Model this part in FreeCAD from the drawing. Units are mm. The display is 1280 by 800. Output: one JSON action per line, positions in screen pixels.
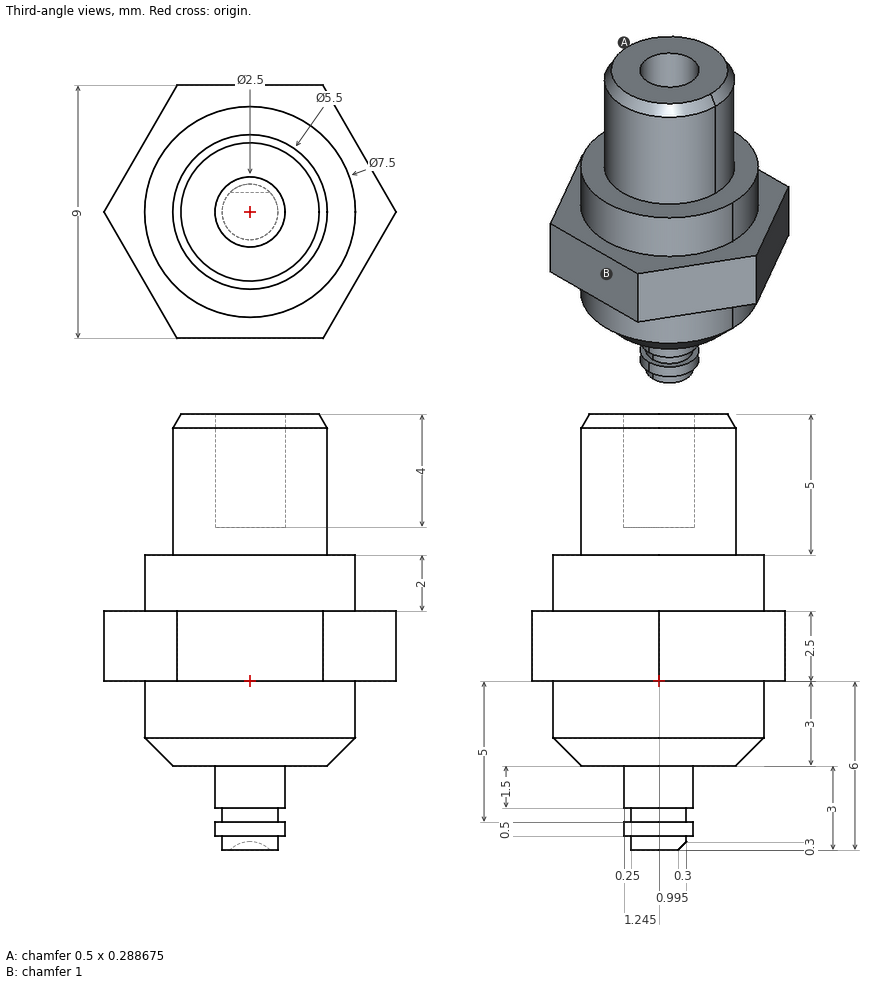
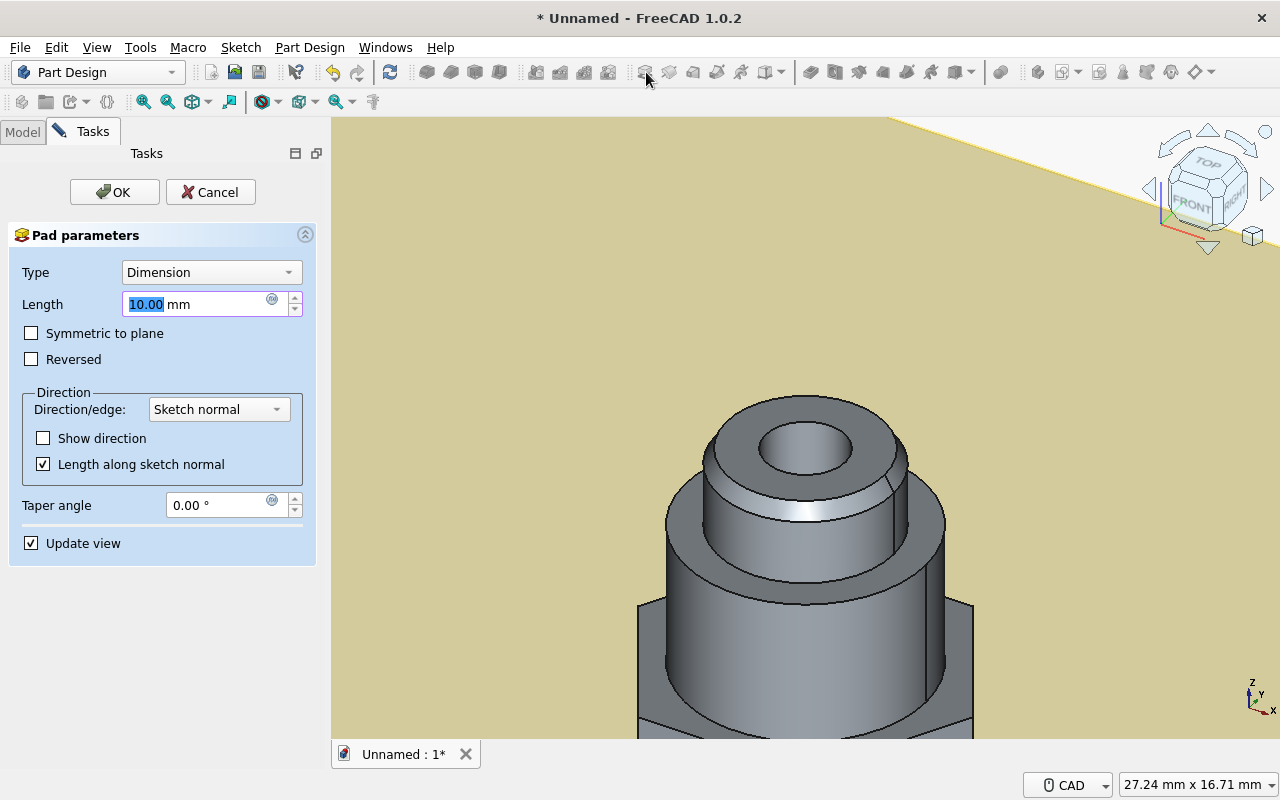
{"action": "type", "text": "3"}
{"action": "key", "text": "Tab"}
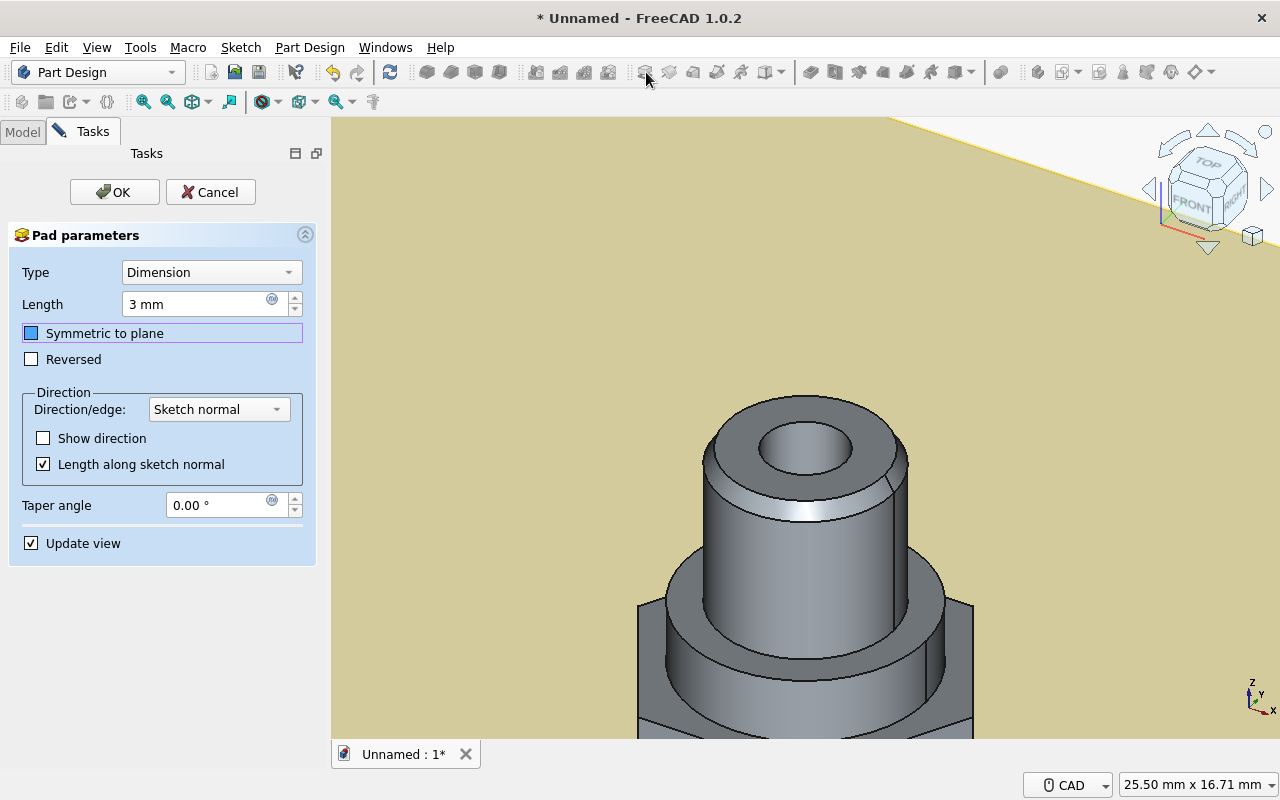
{"action": "left_click", "coordinate": [115, 192]}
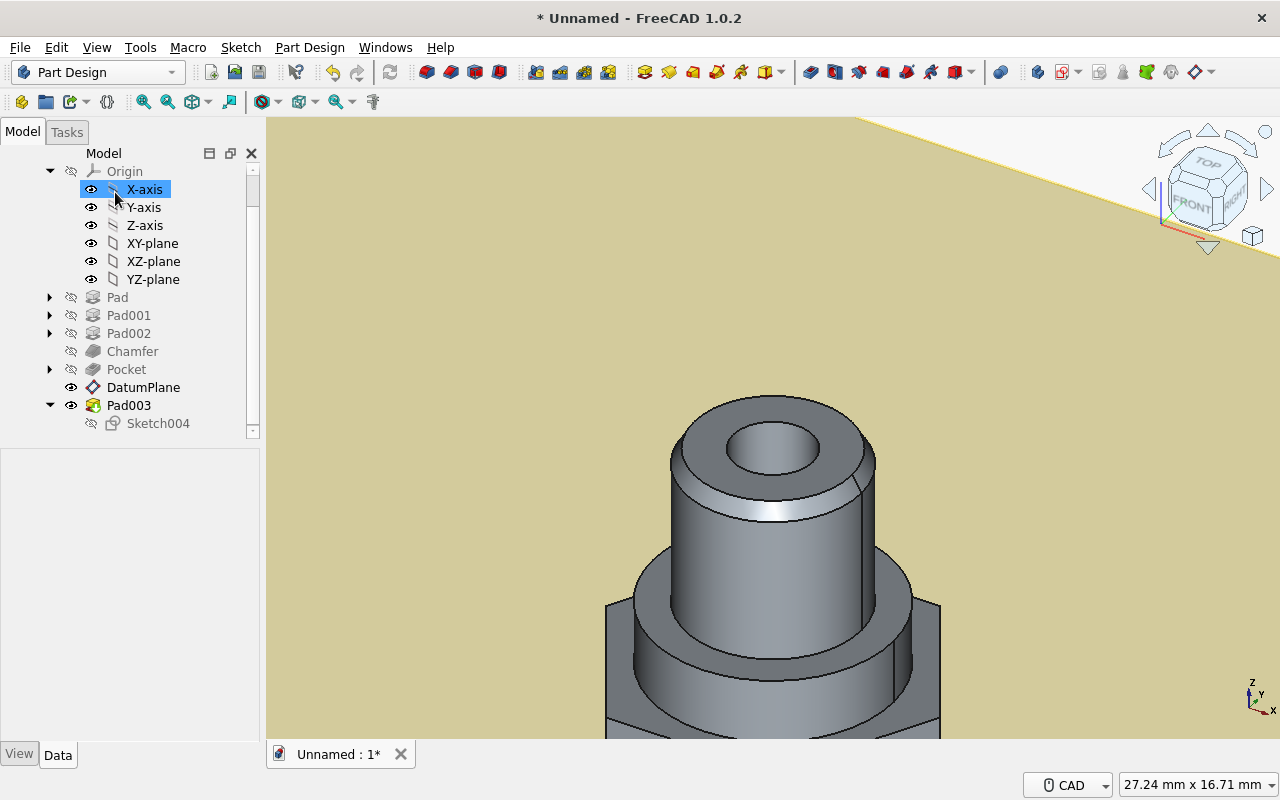
{"action": "left_click", "coordinate": [116, 387]}
{"action": "key", "text": "space"}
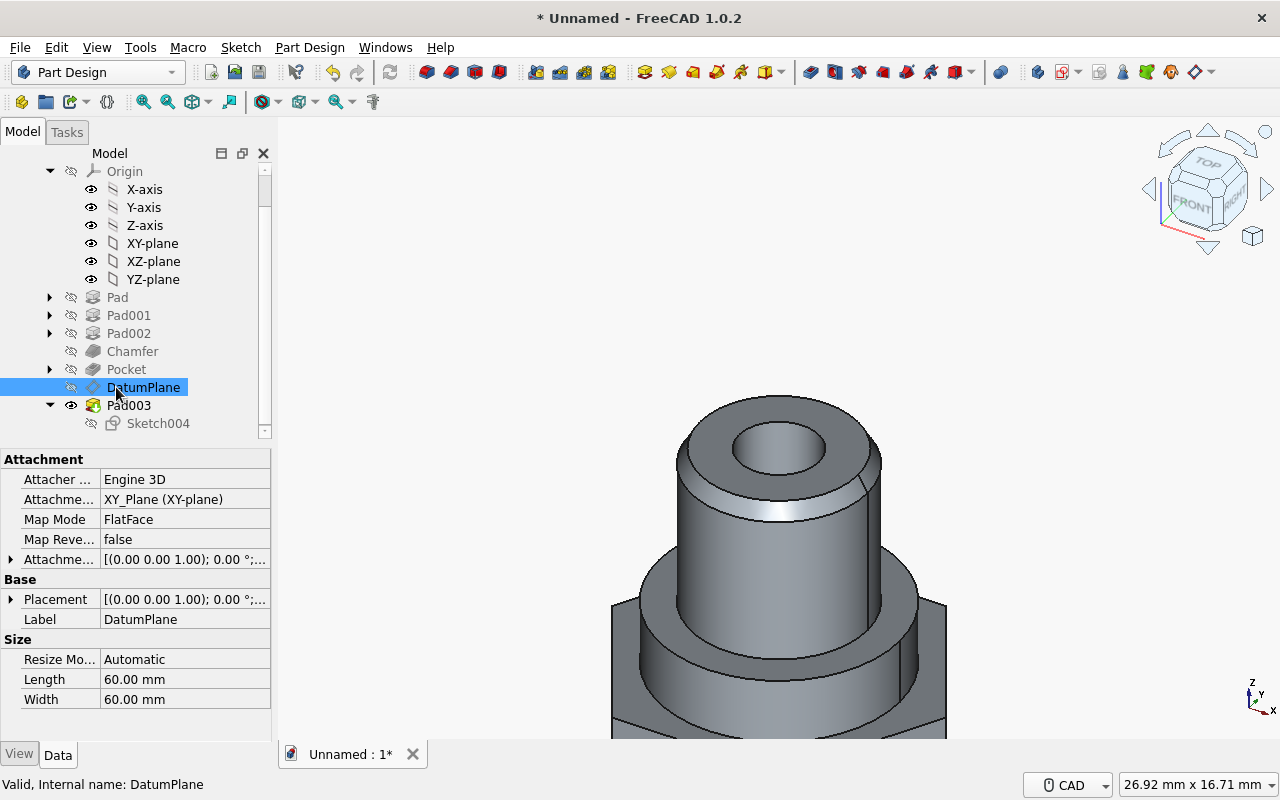
{"action": "key", "text": "v f"}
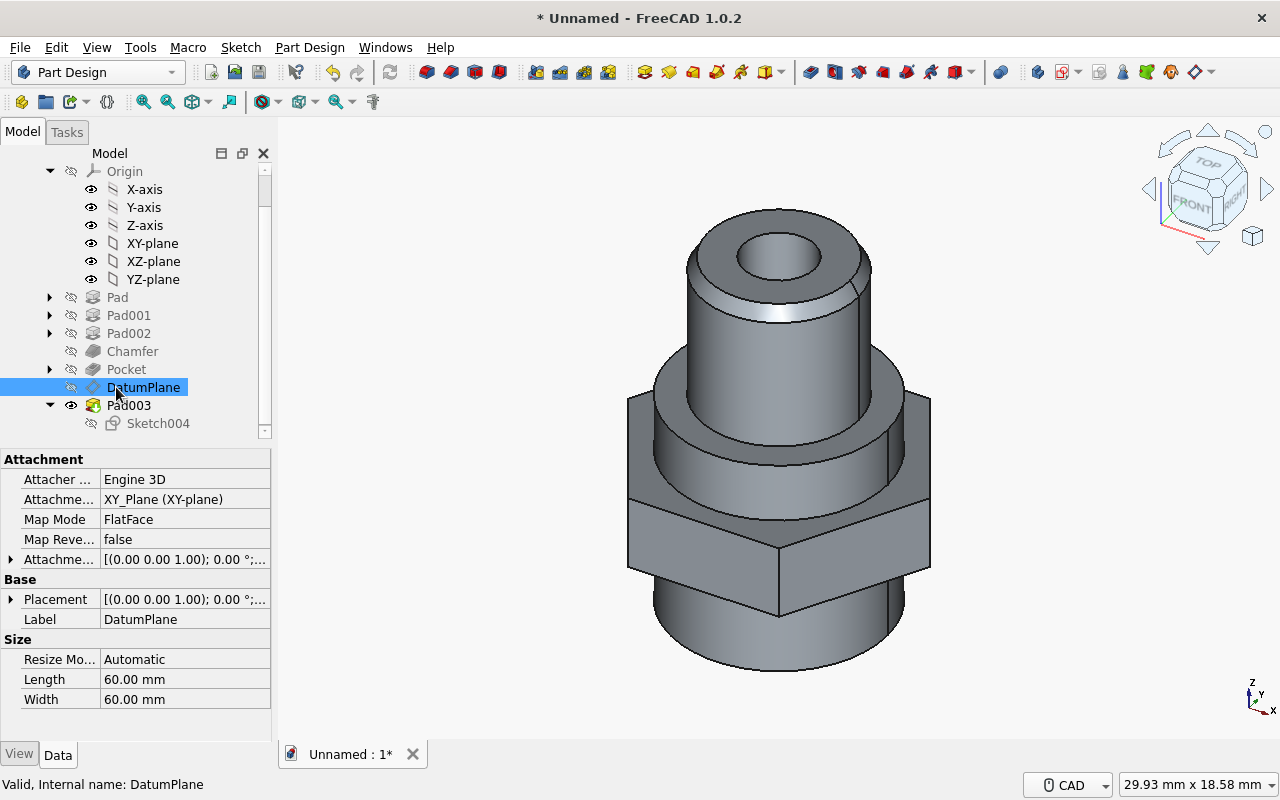
{"action": "key", "text": "0"}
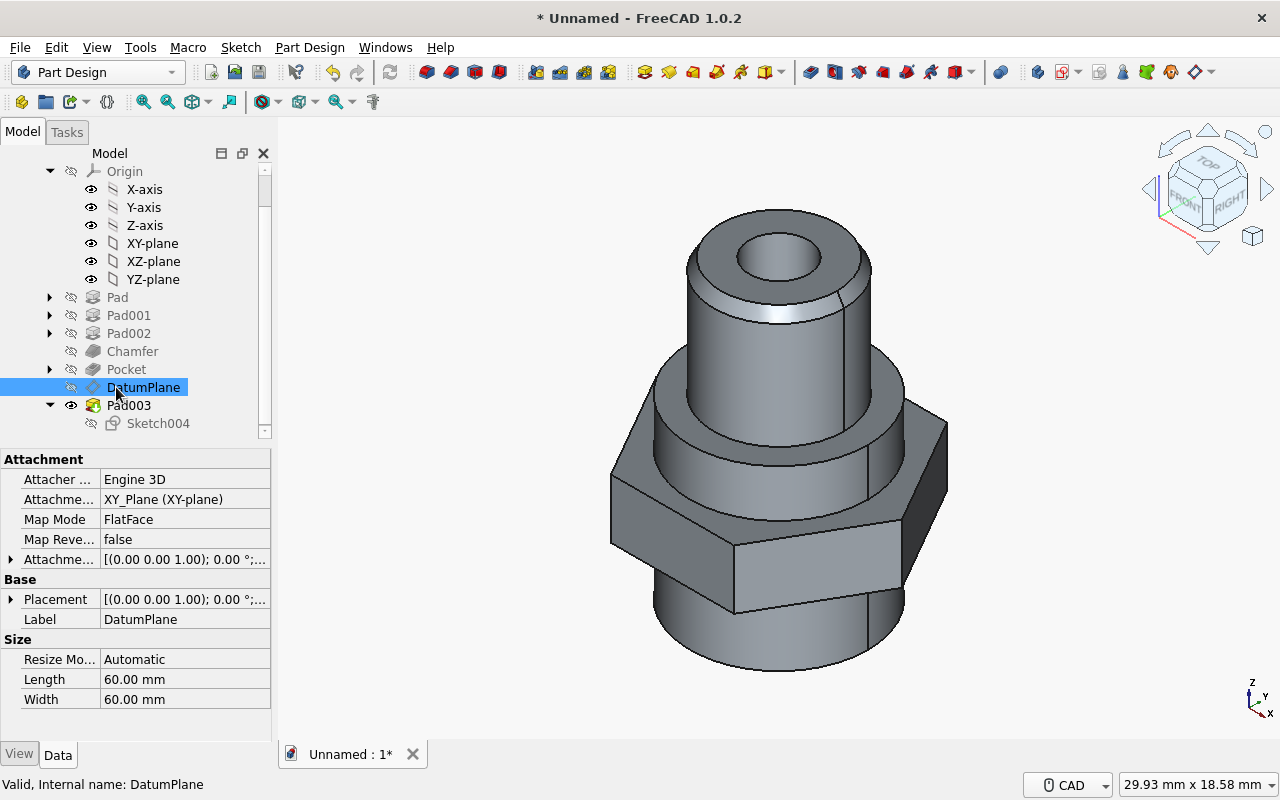
{"action": "left_click", "coordinate": [883, 639]}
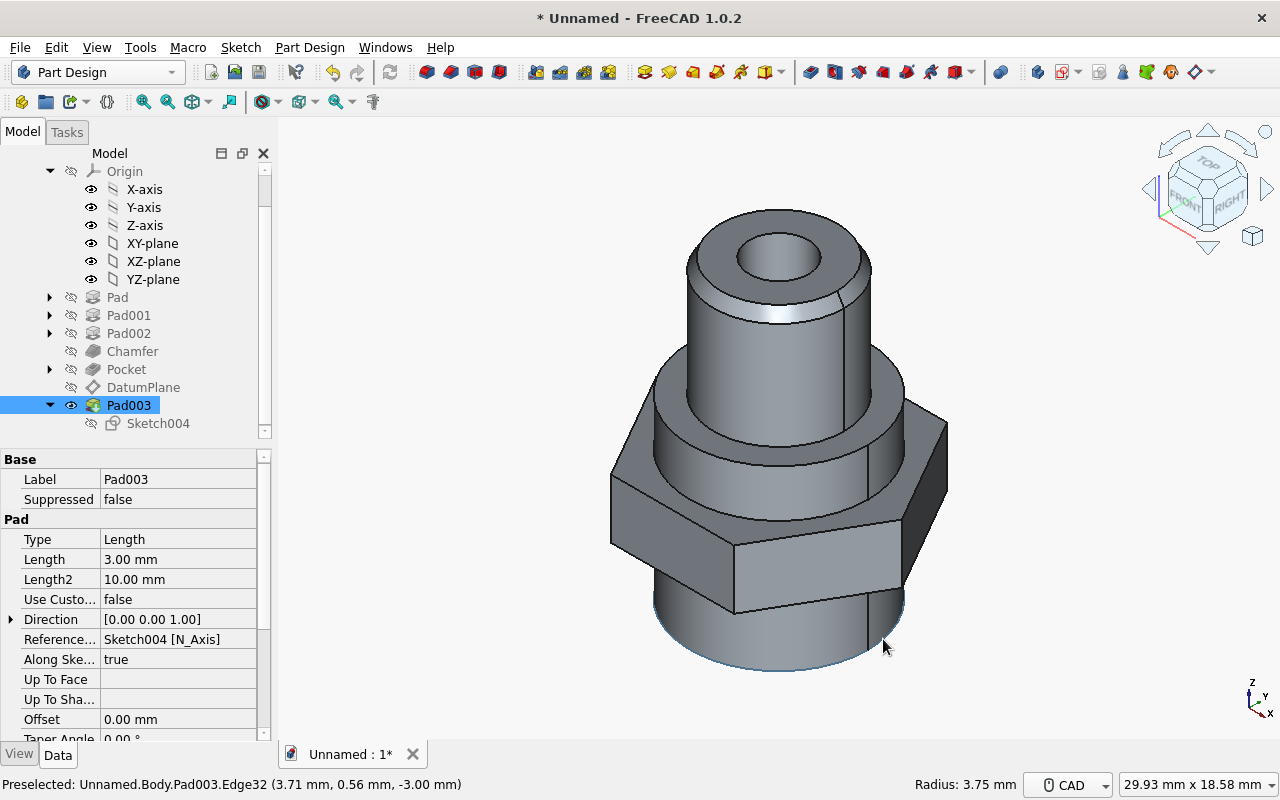
{"action": "left_click", "coordinate": [452, 72]}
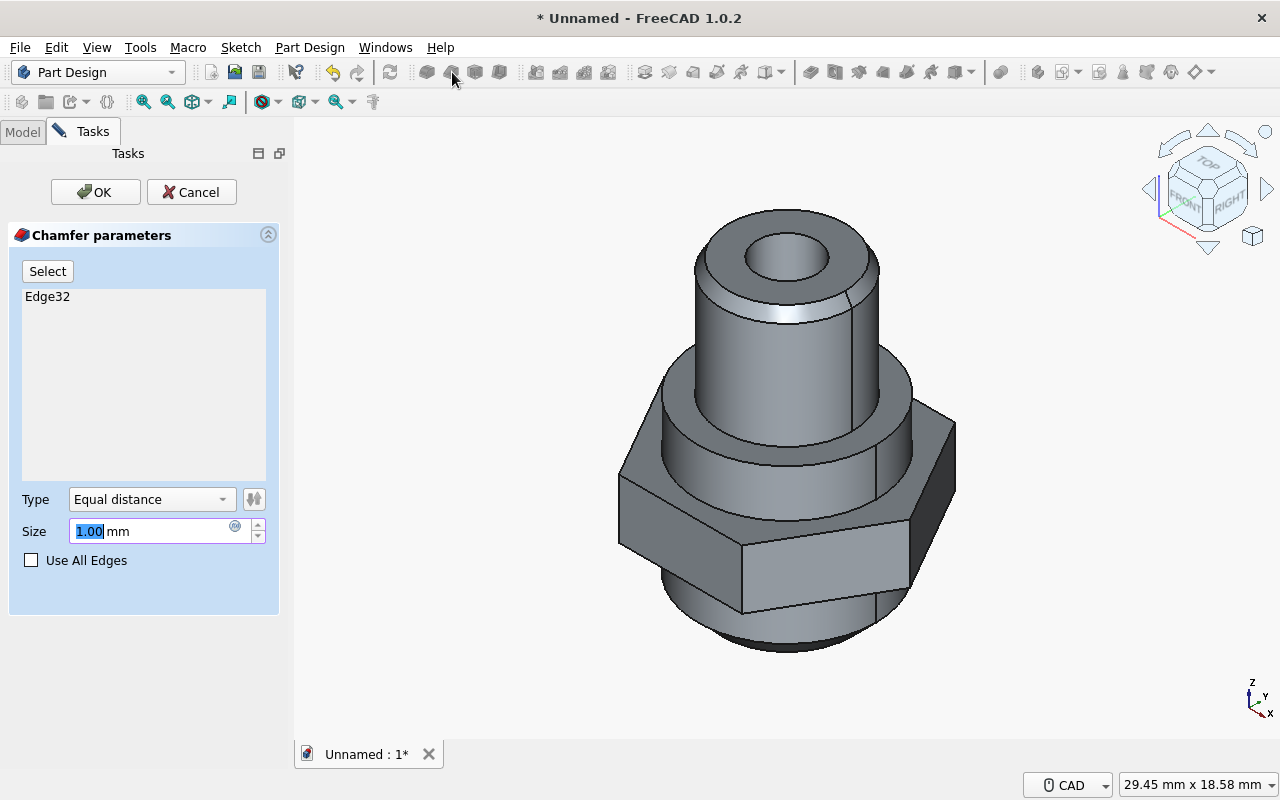
{"action": "type", "text": "1"}
{"action": "key", "text": "Tab"}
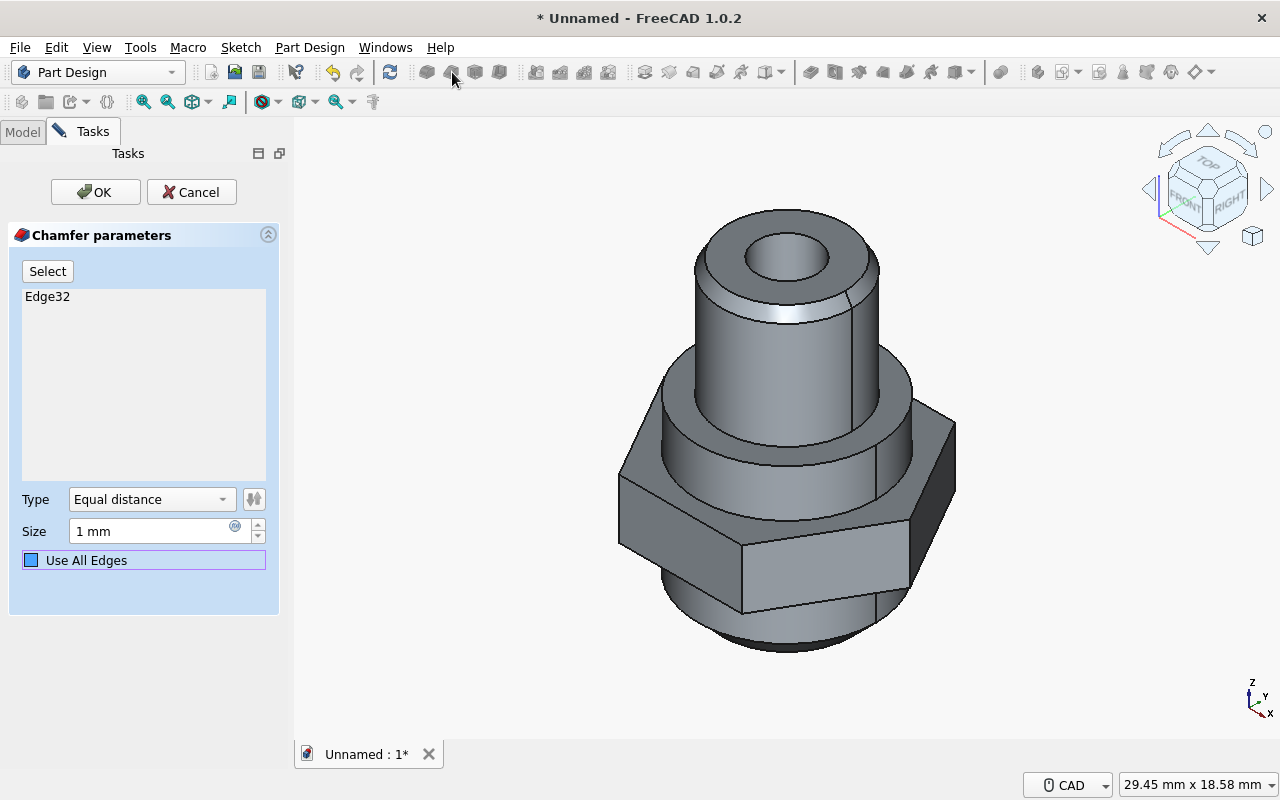
{"action": "left_click", "coordinate": [96, 192]}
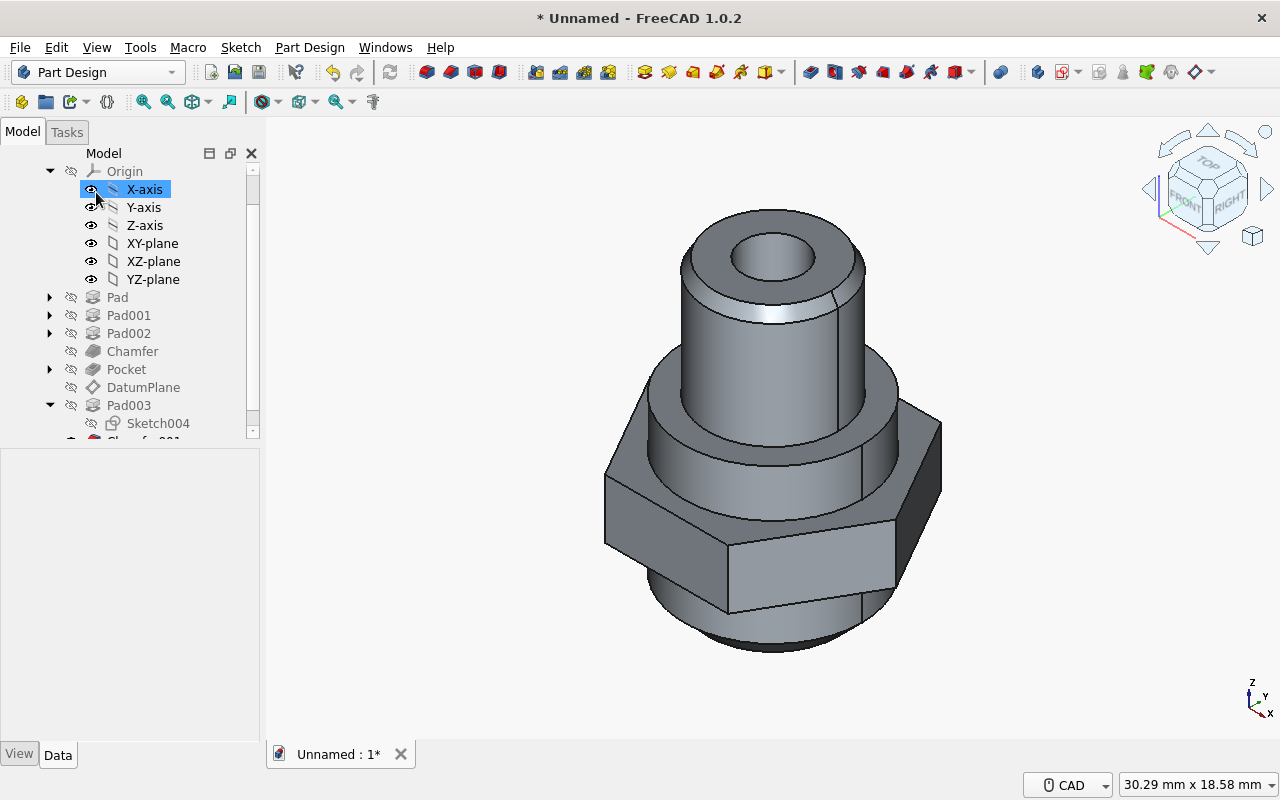
{"action": "left_click", "coordinate": [1062, 72]}